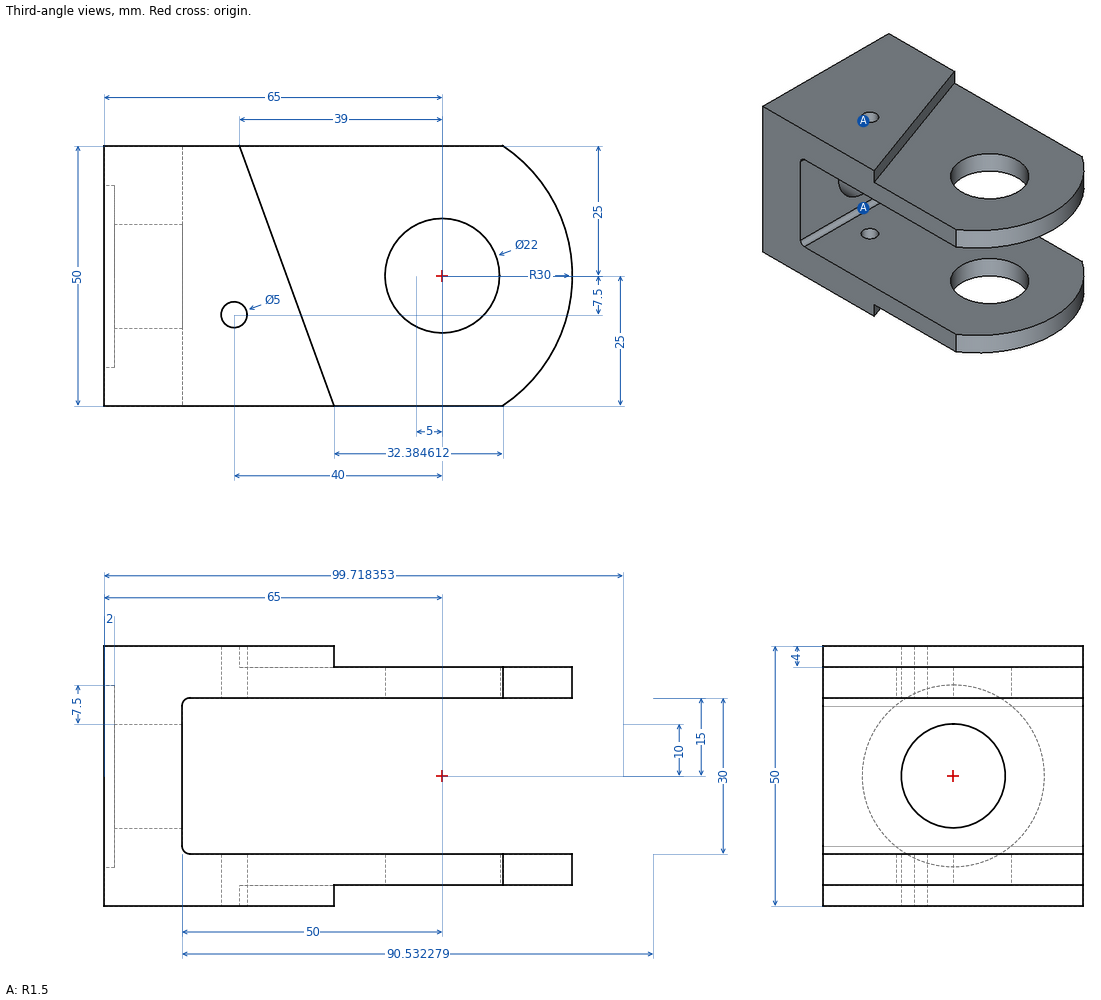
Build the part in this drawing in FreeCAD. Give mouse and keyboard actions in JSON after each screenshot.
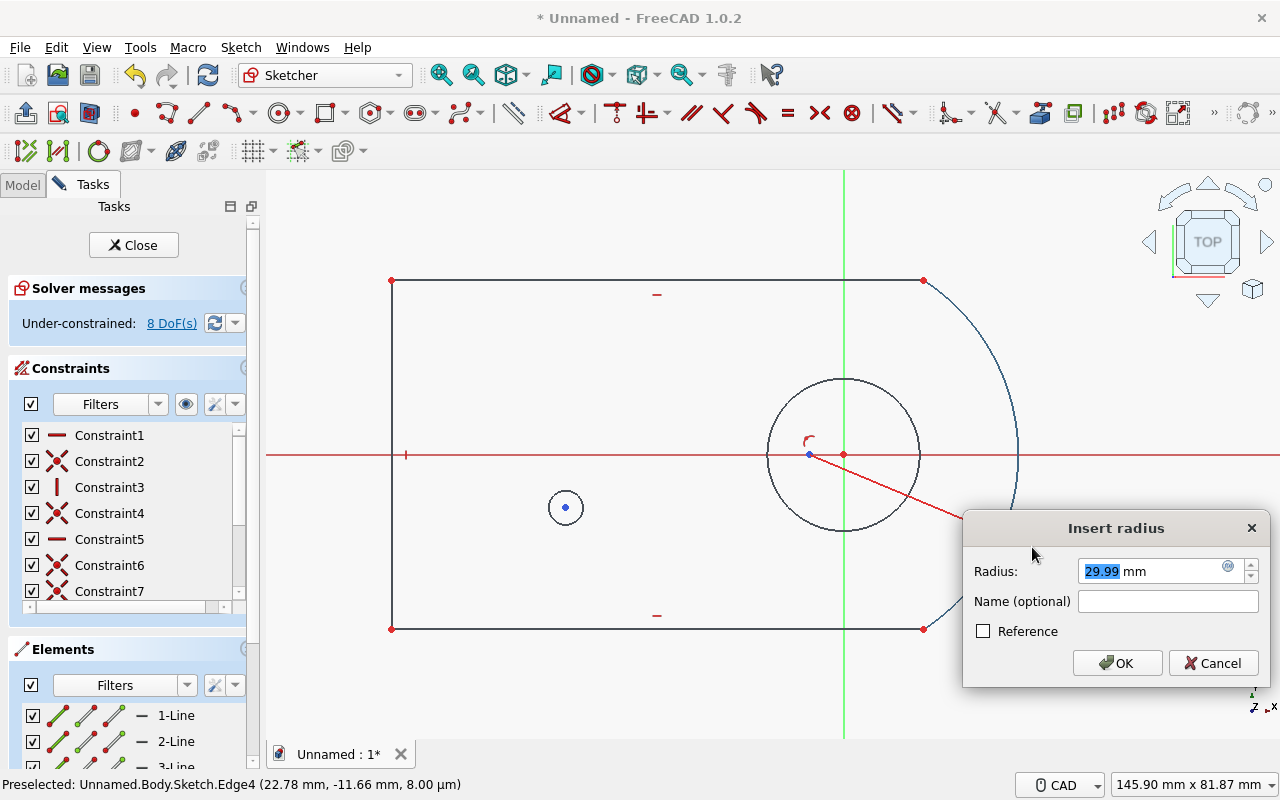
{"action": "type", "text": "30"}
{"action": "key", "text": "Return"}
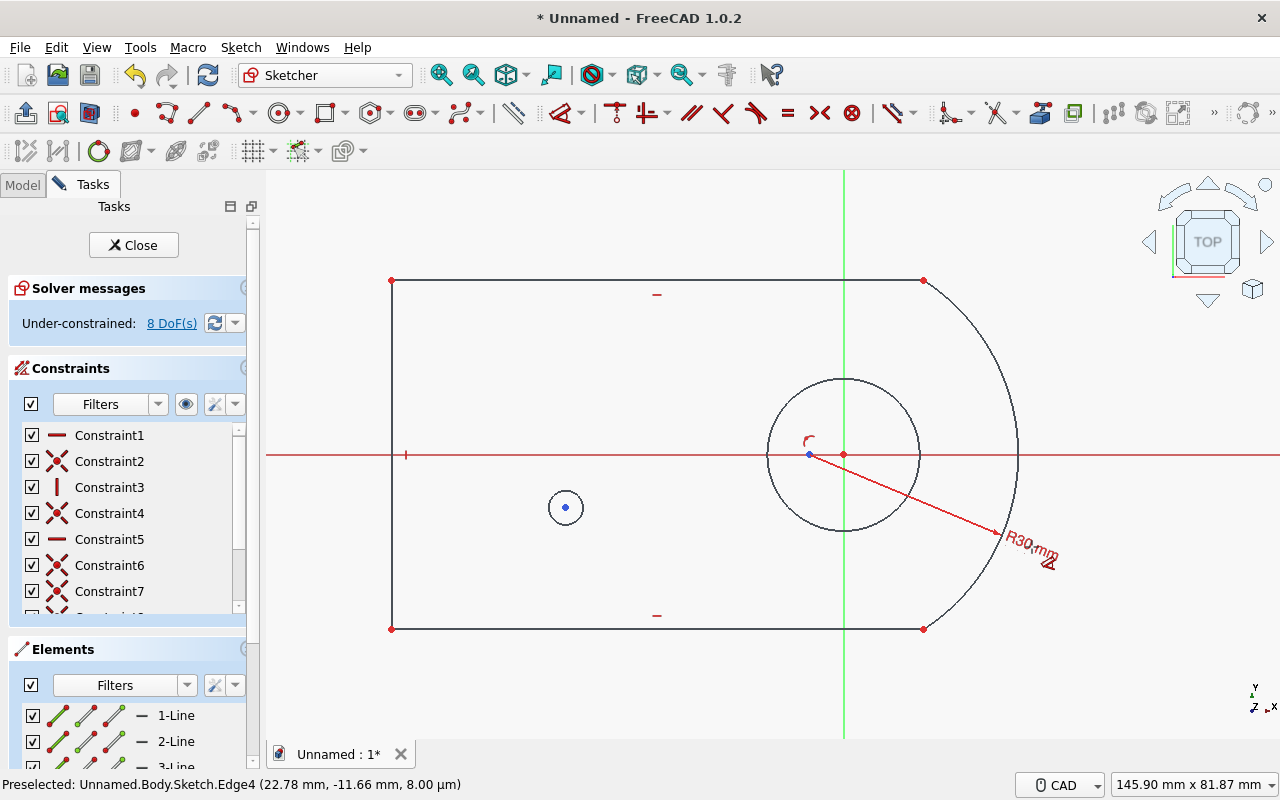
{"action": "left_click", "coordinate": [578, 496]}
{"action": "left_click", "coordinate": [601, 474]}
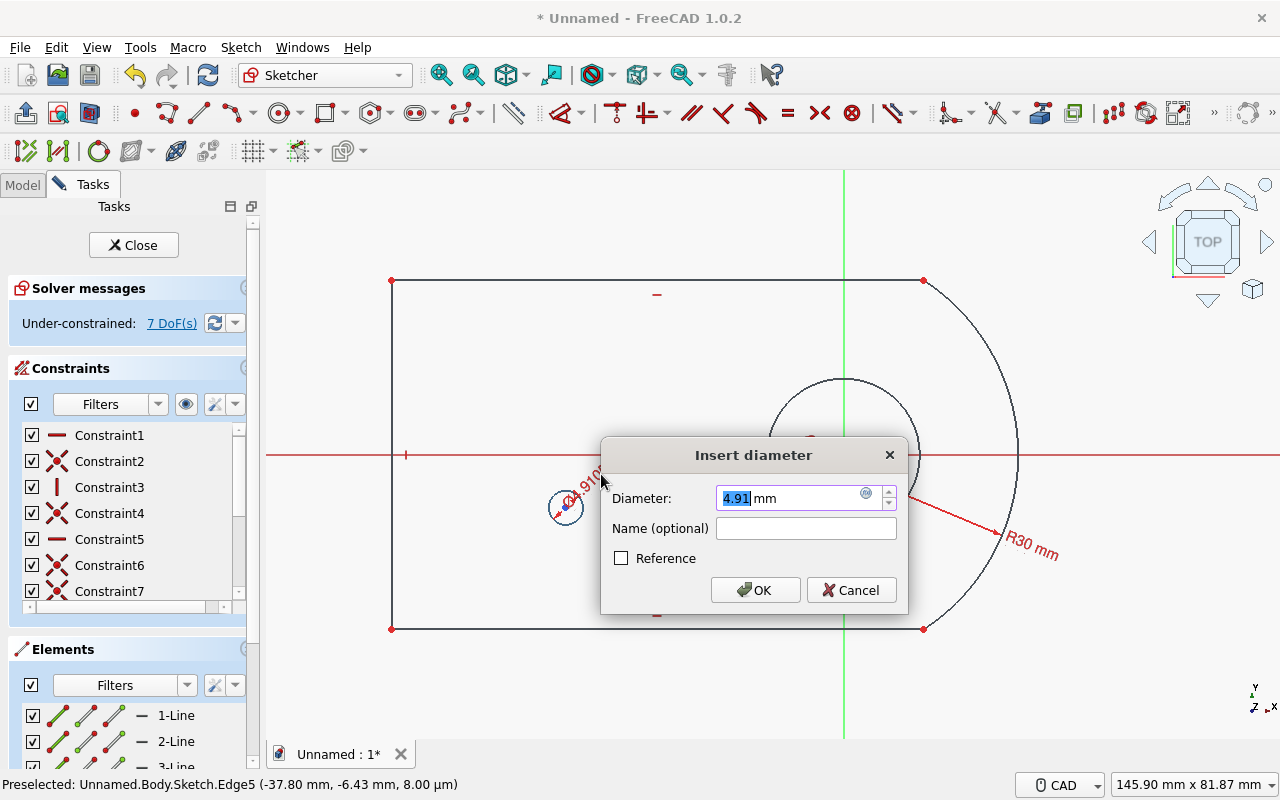
{"action": "type", "text": "5"}
{"action": "key", "text": "Return"}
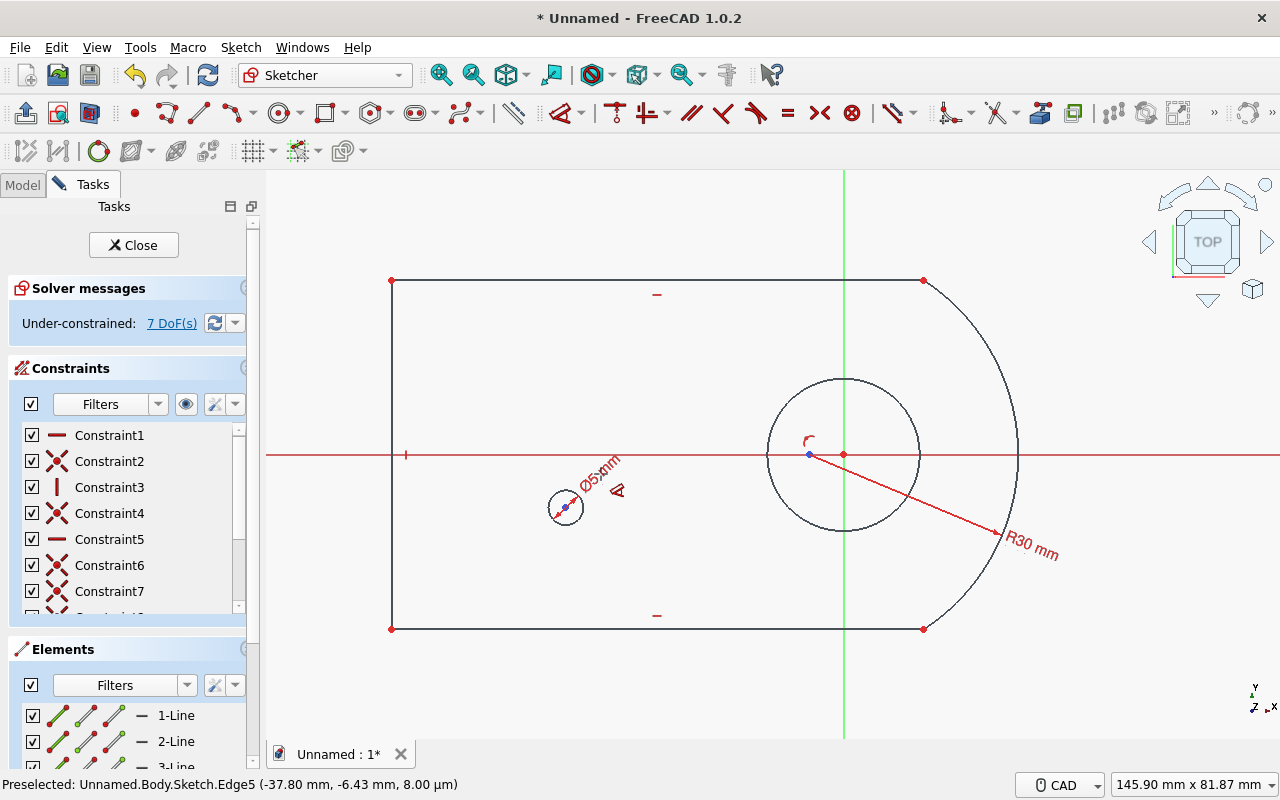
{"action": "left_click", "coordinate": [897, 401]}
{"action": "left_click", "coordinate": [920, 378]}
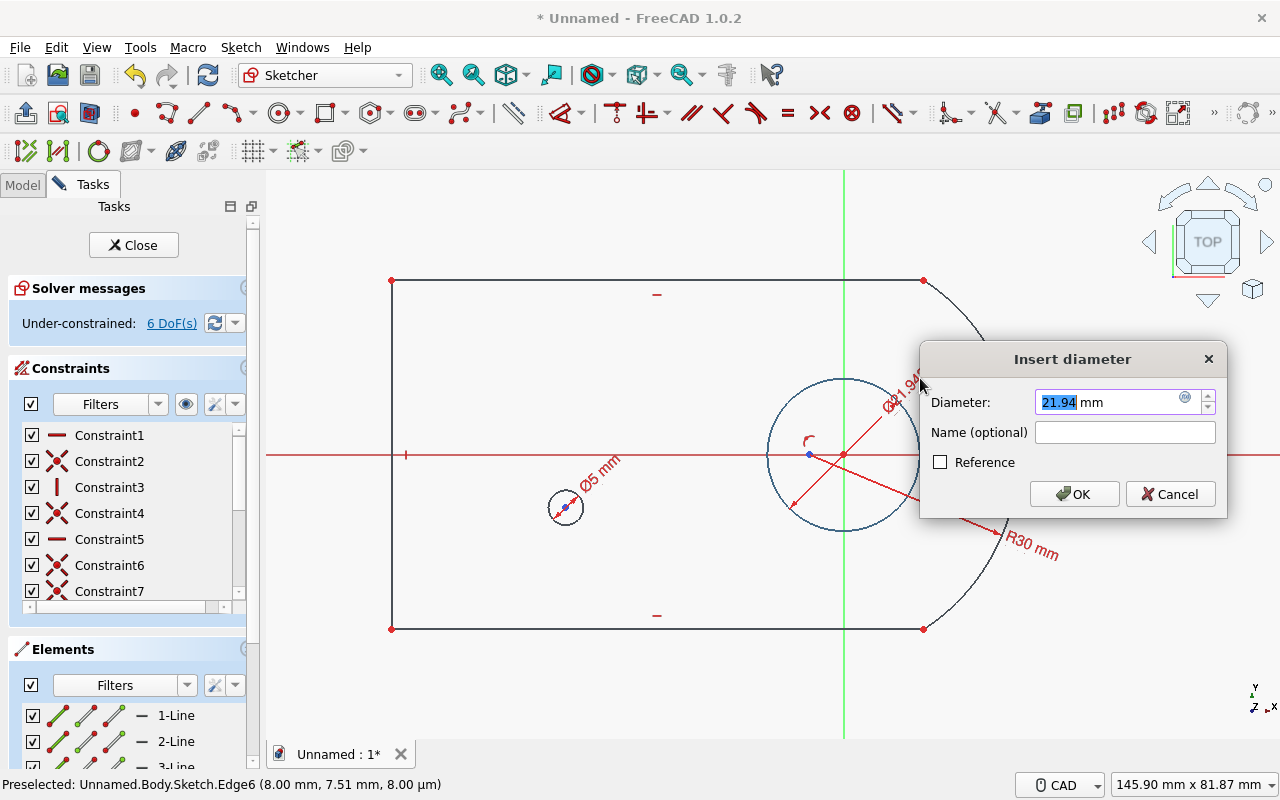
{"action": "type", "text": "22"}
{"action": "key", "text": "Return"}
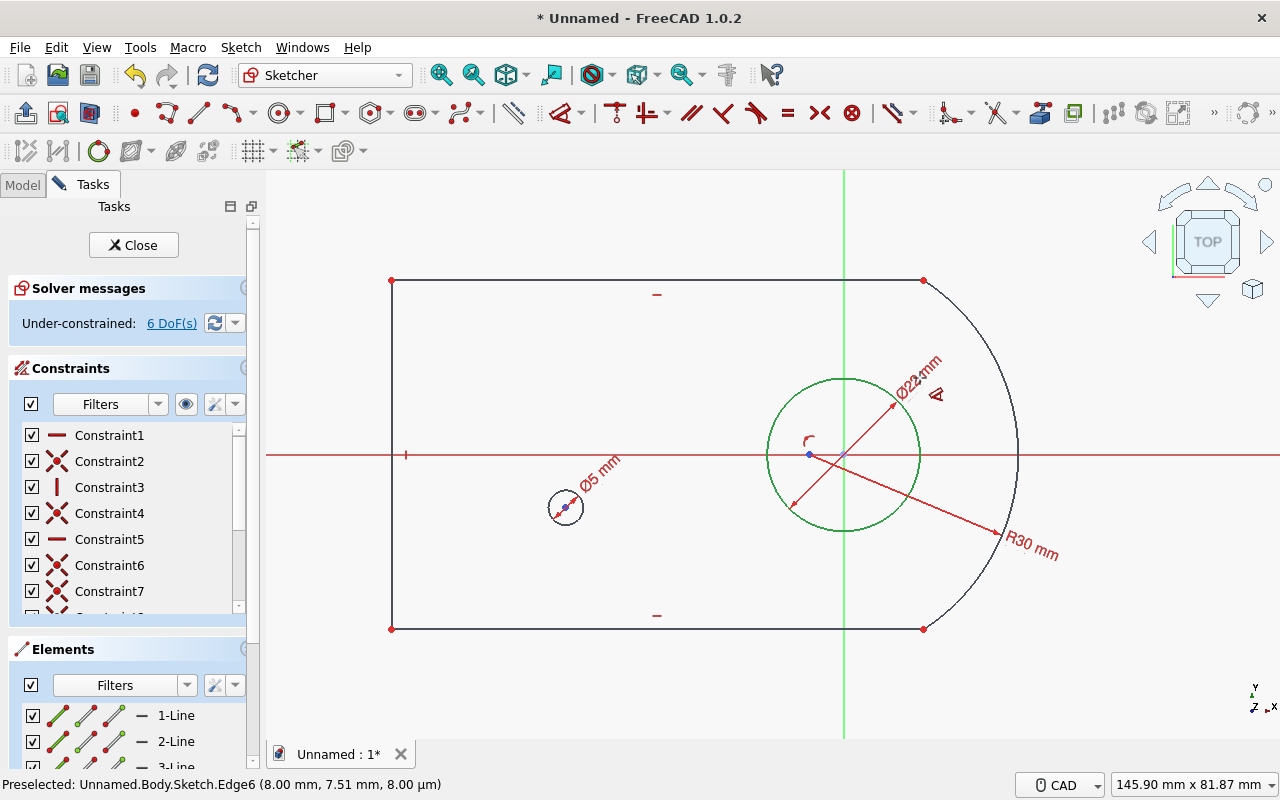
{"action": "left_click", "coordinate": [392, 385]}
{"action": "left_click", "coordinate": [358, 375]}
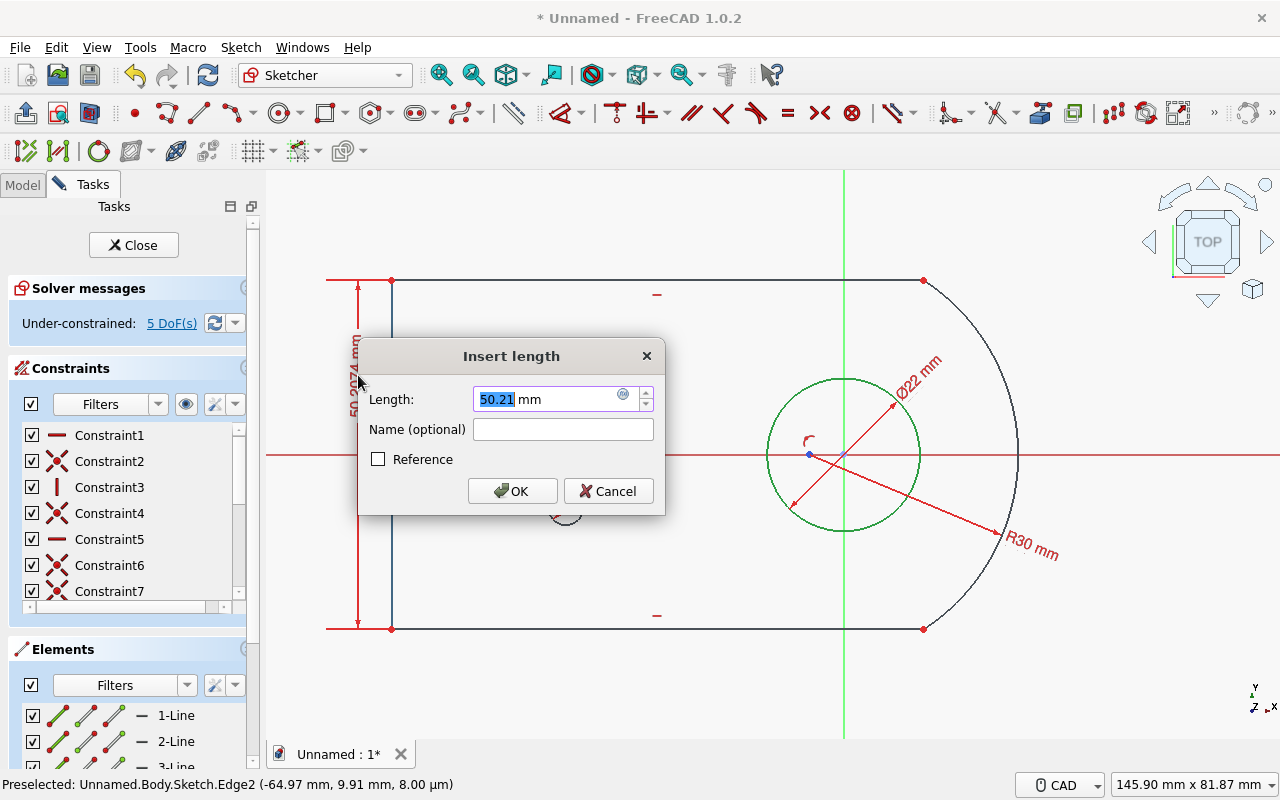
{"action": "type", "text": "50"}
{"action": "key", "text": "Return"}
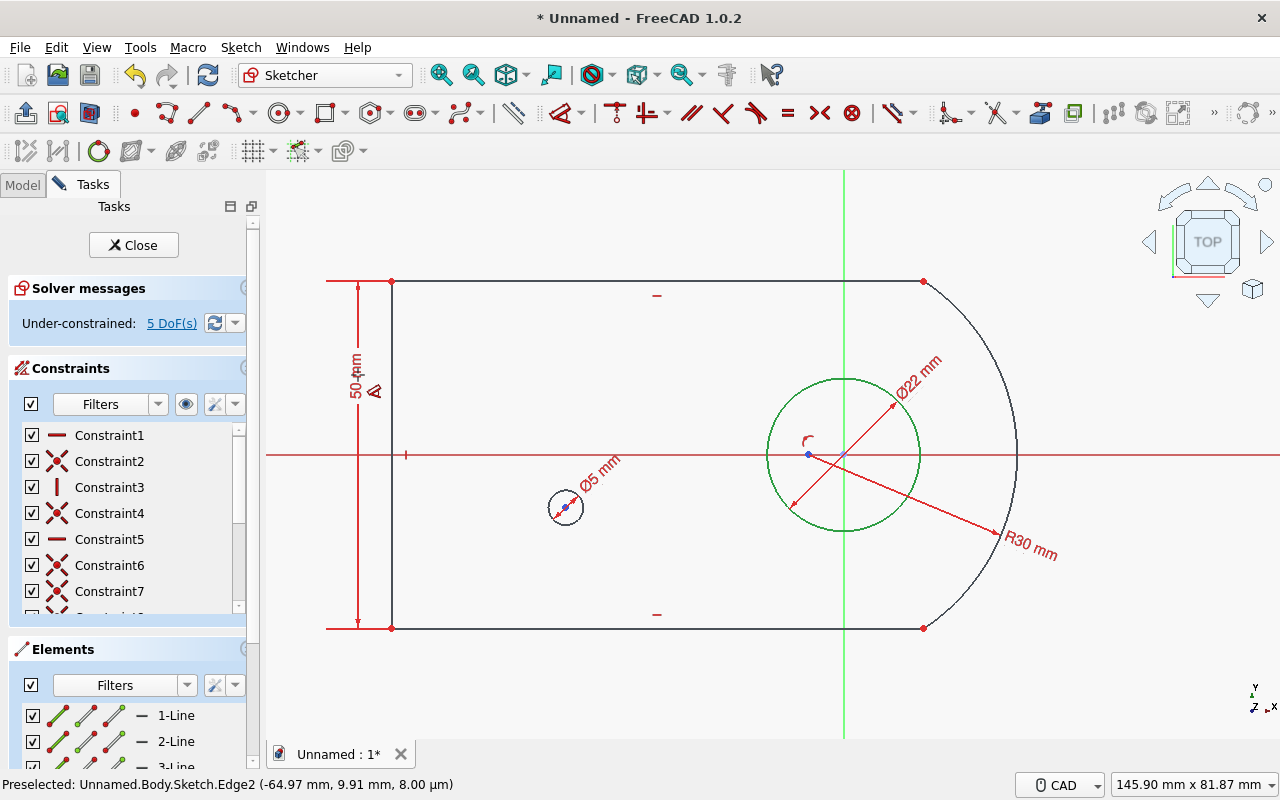
{"action": "left_click", "coordinate": [809, 455]}
{"action": "left_click", "coordinate": [826, 489]}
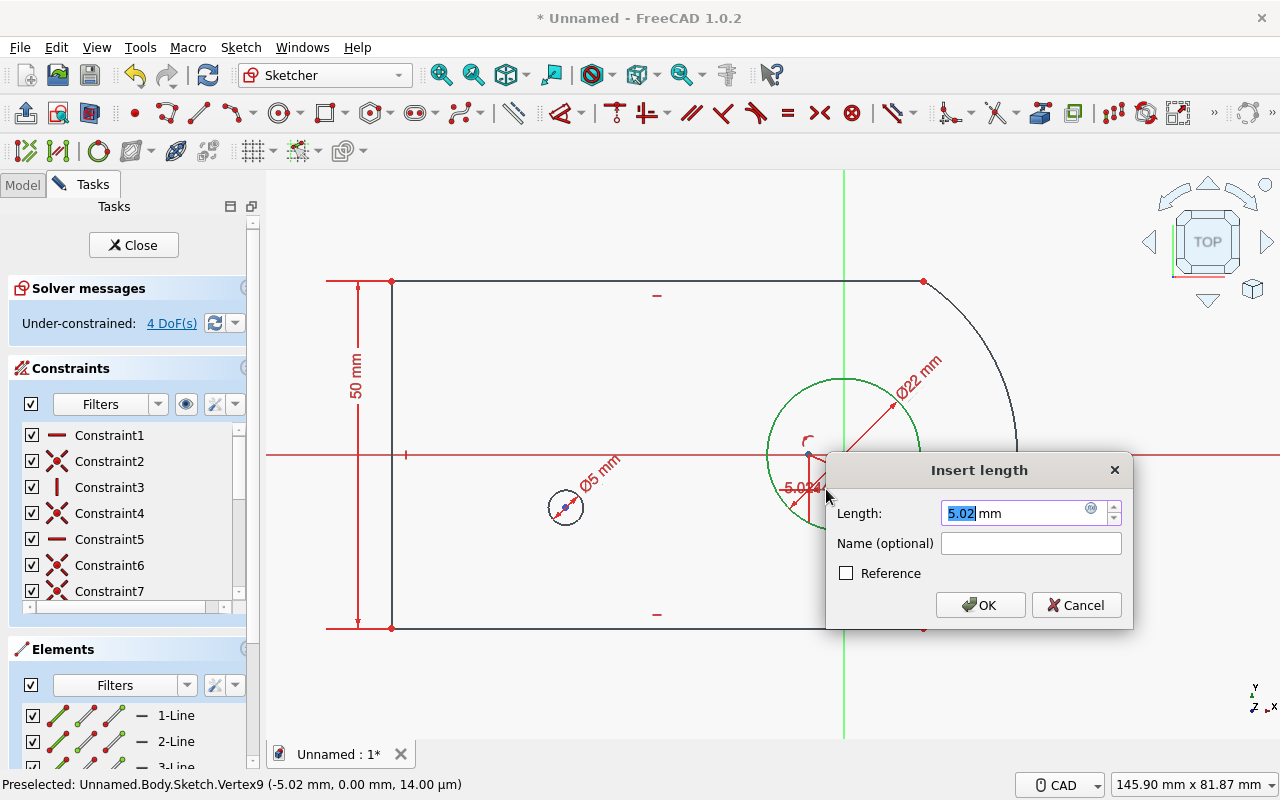
{"action": "type", "text": "5"}
{"action": "key", "text": "Return"}